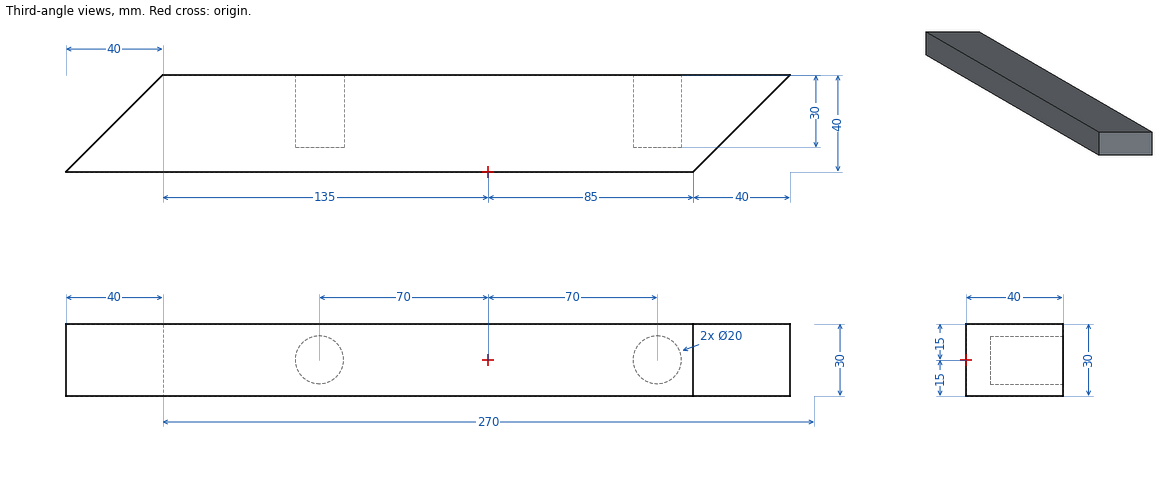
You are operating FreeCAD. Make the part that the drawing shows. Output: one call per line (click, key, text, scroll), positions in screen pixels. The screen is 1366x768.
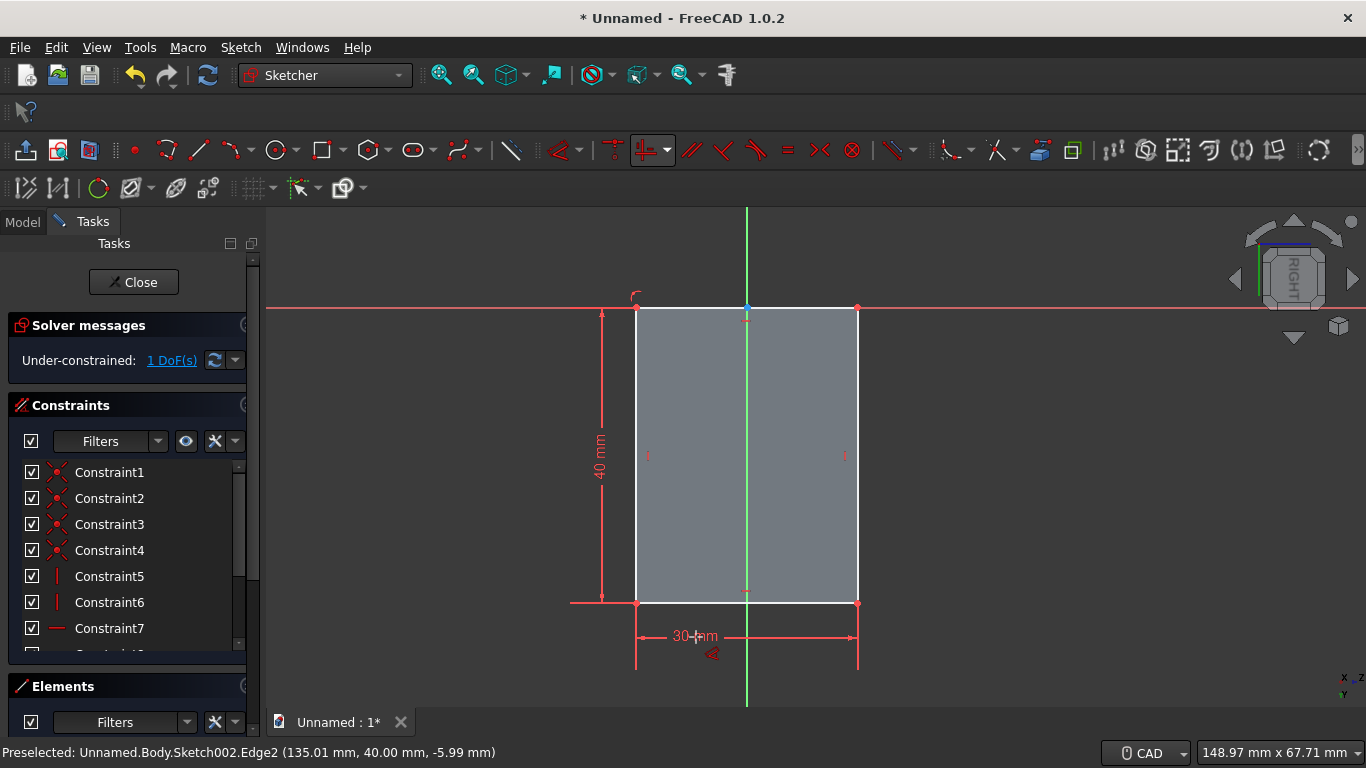
click(636, 308)
click(692, 274)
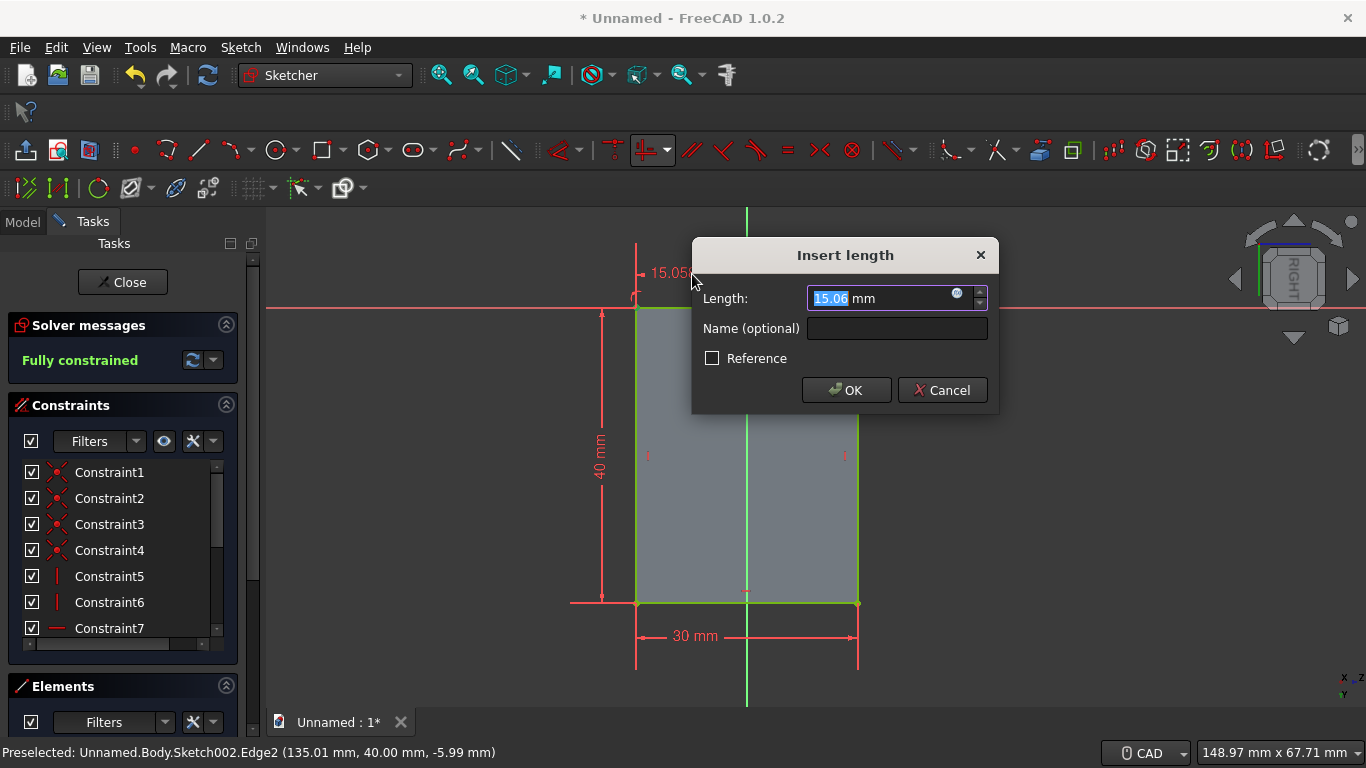
text(15)
key(Return)
key(Escape)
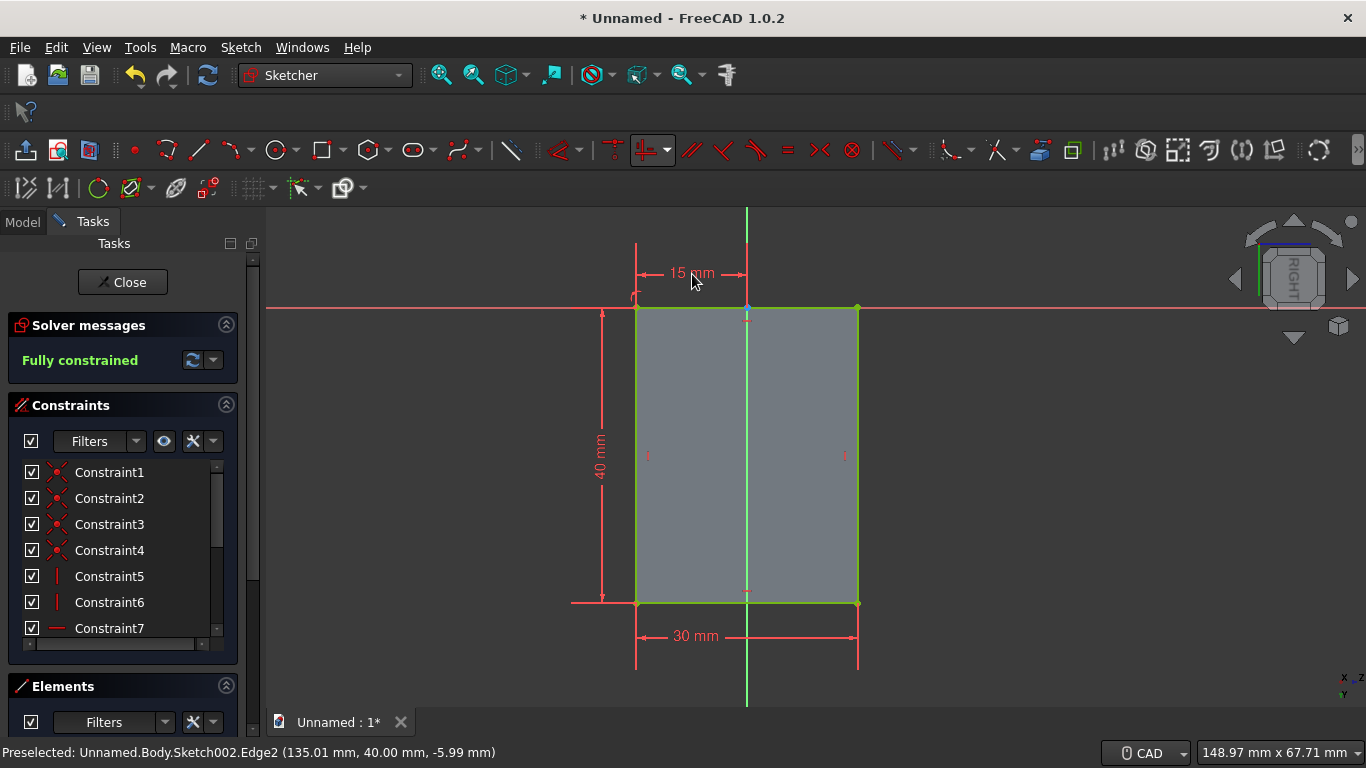
click(123, 282)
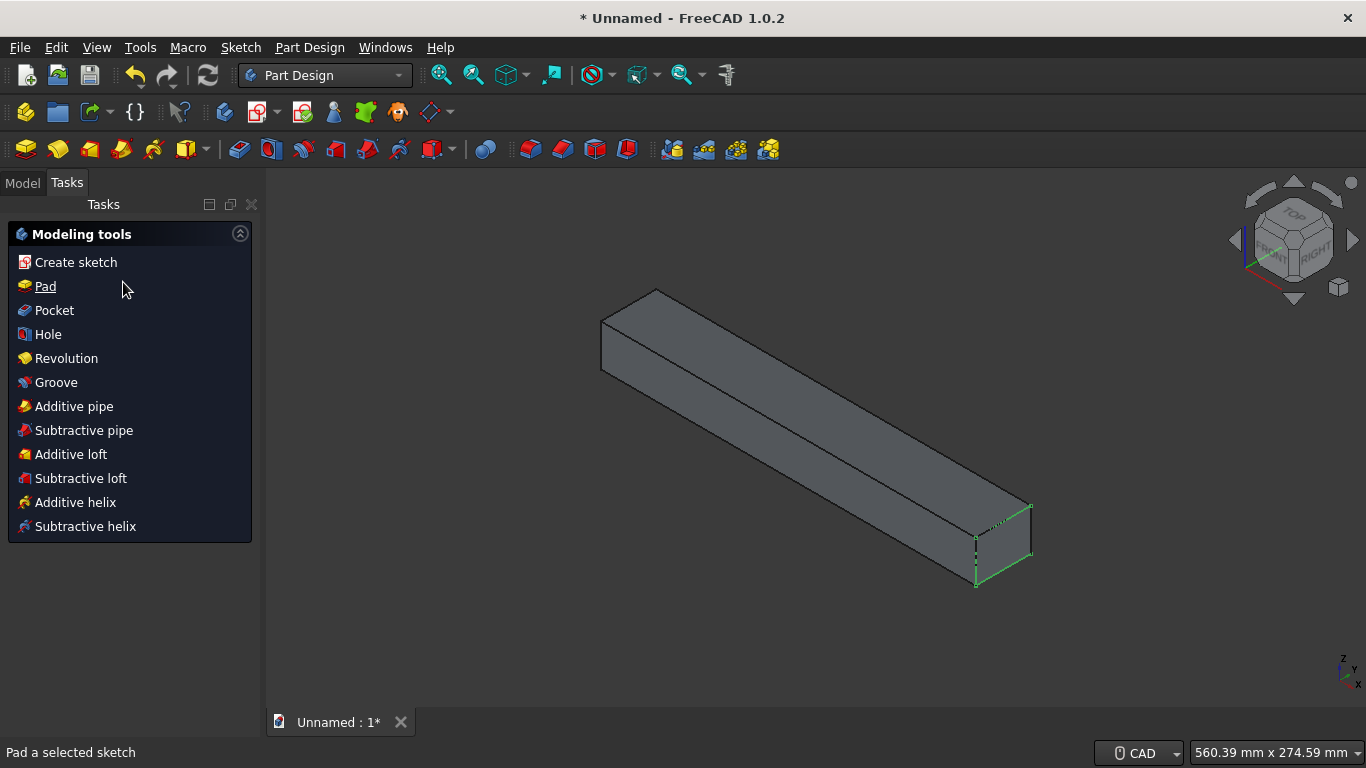
click(240, 150)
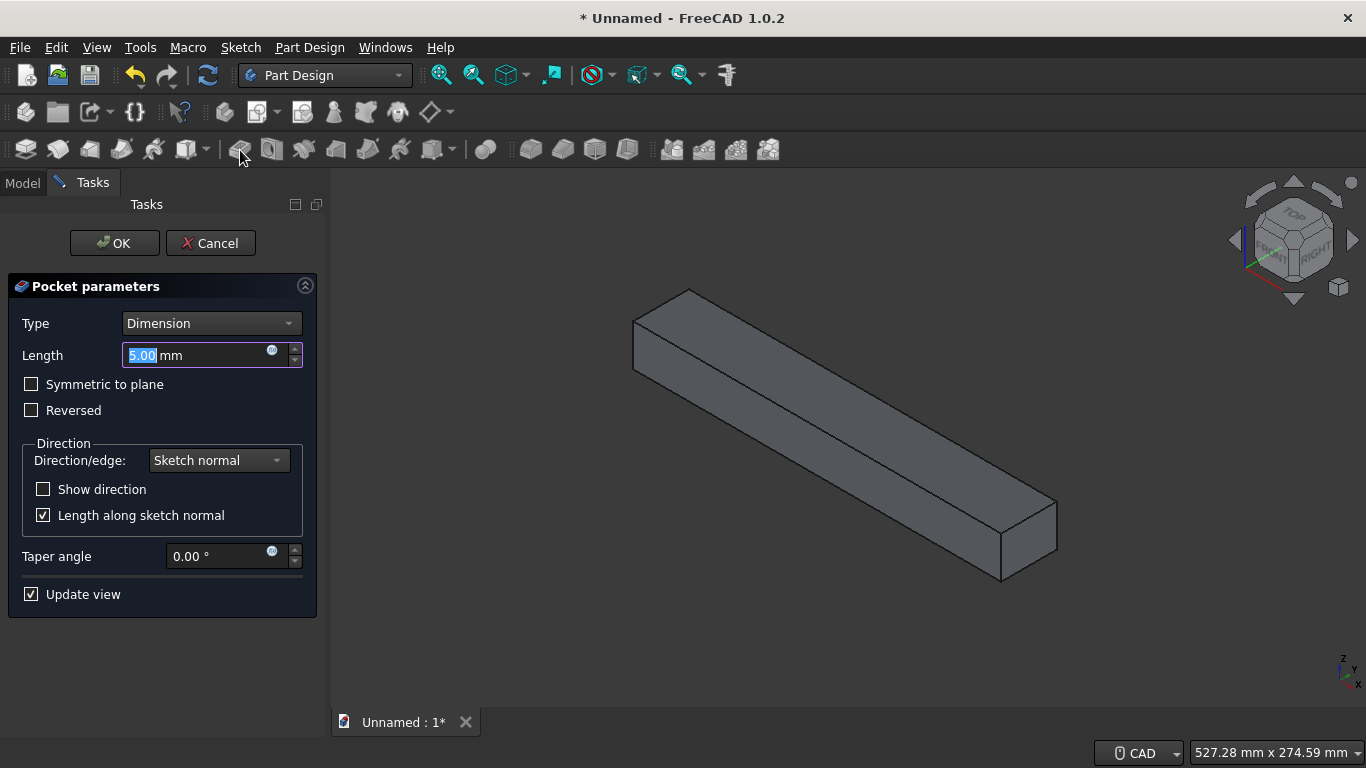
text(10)
key(Tab)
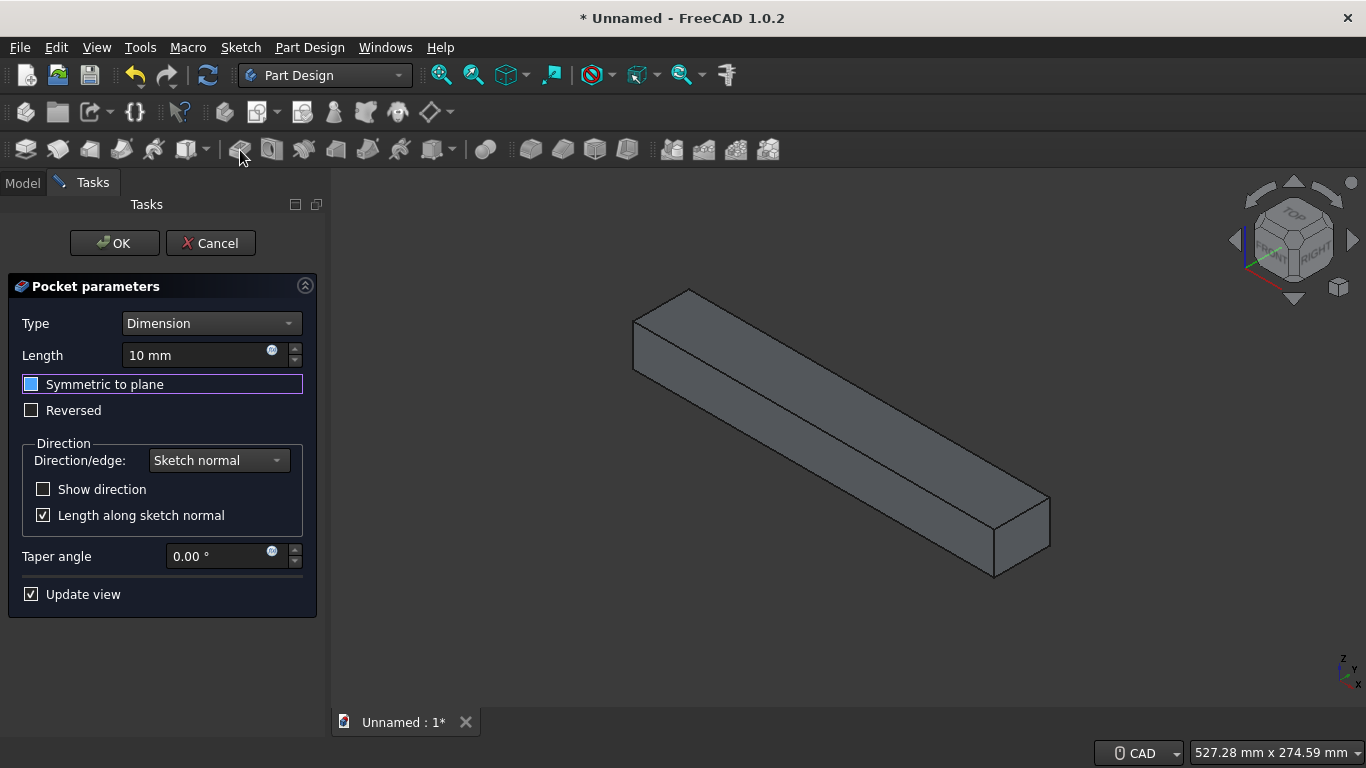
click(115, 243)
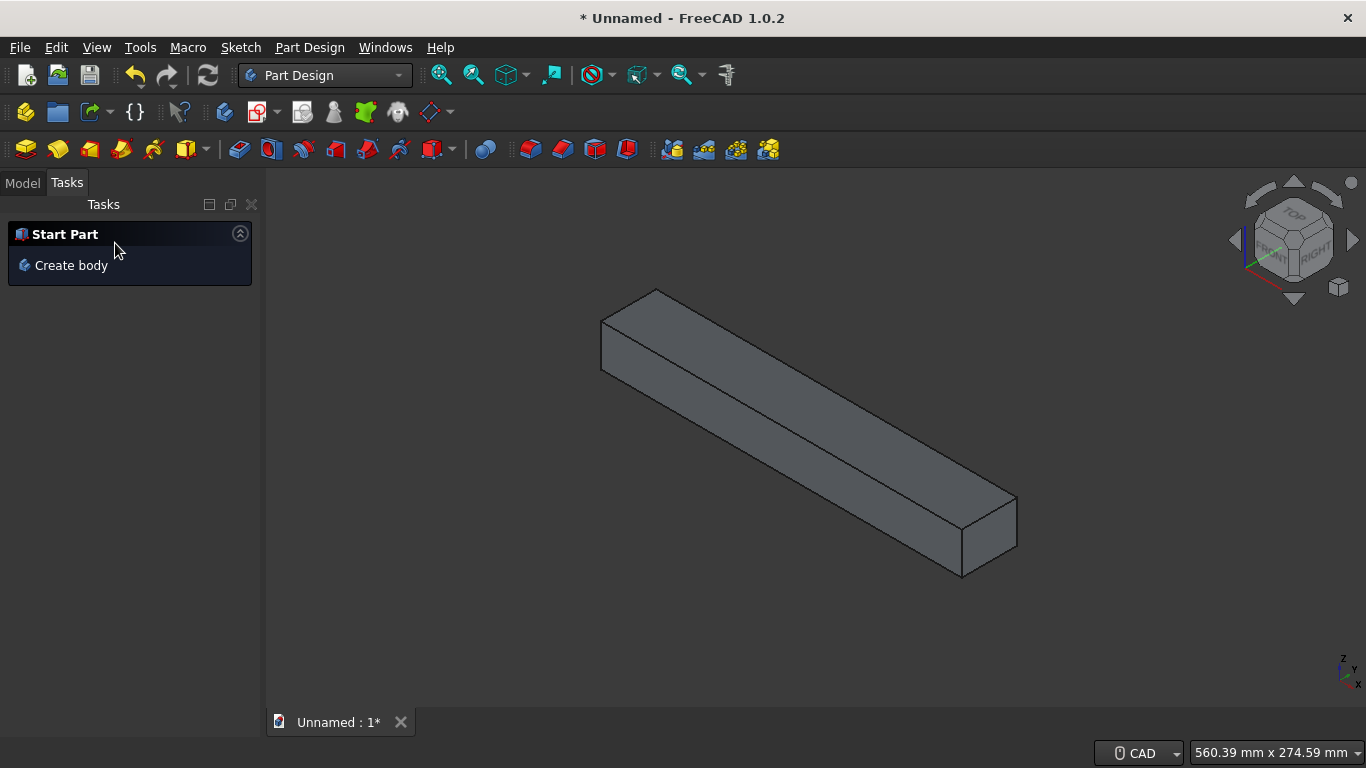
click(912, 468)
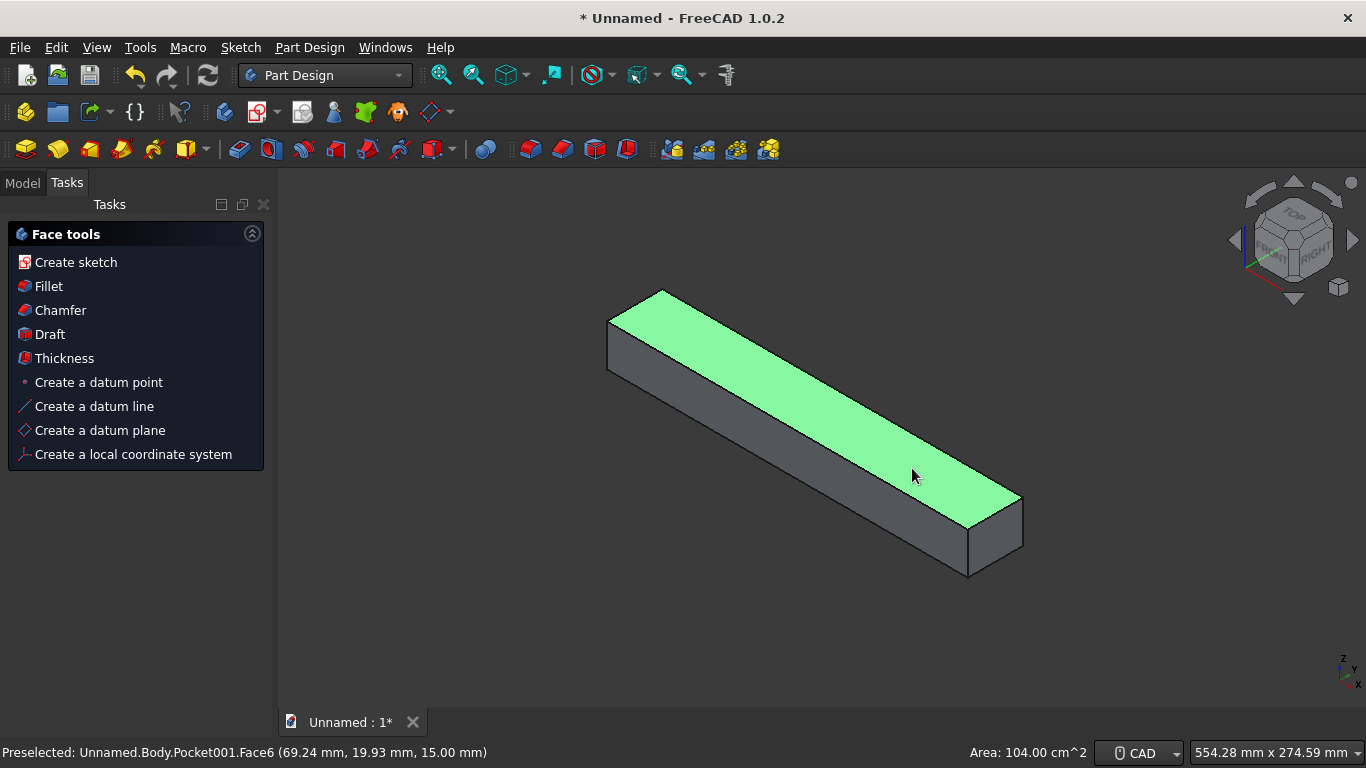
click(258, 112)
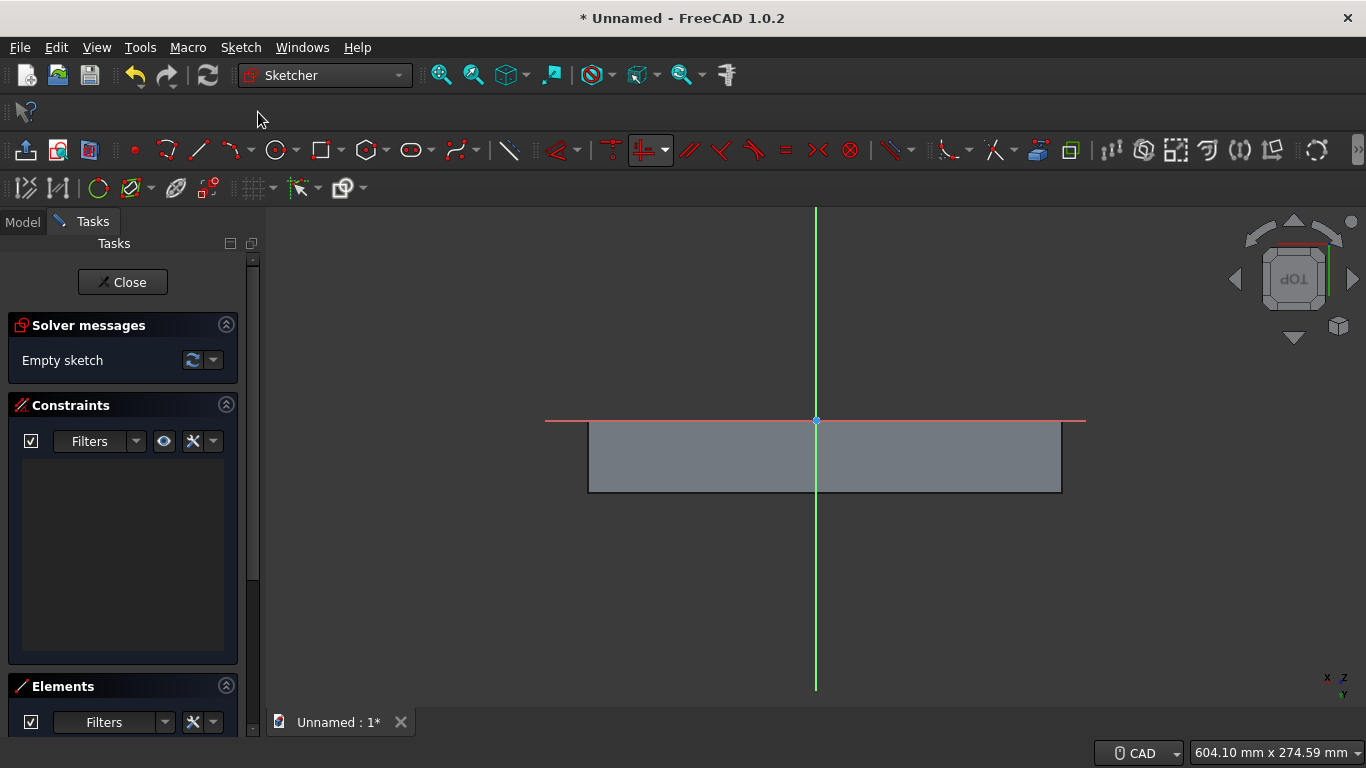
scroll(585, 457, up, 7)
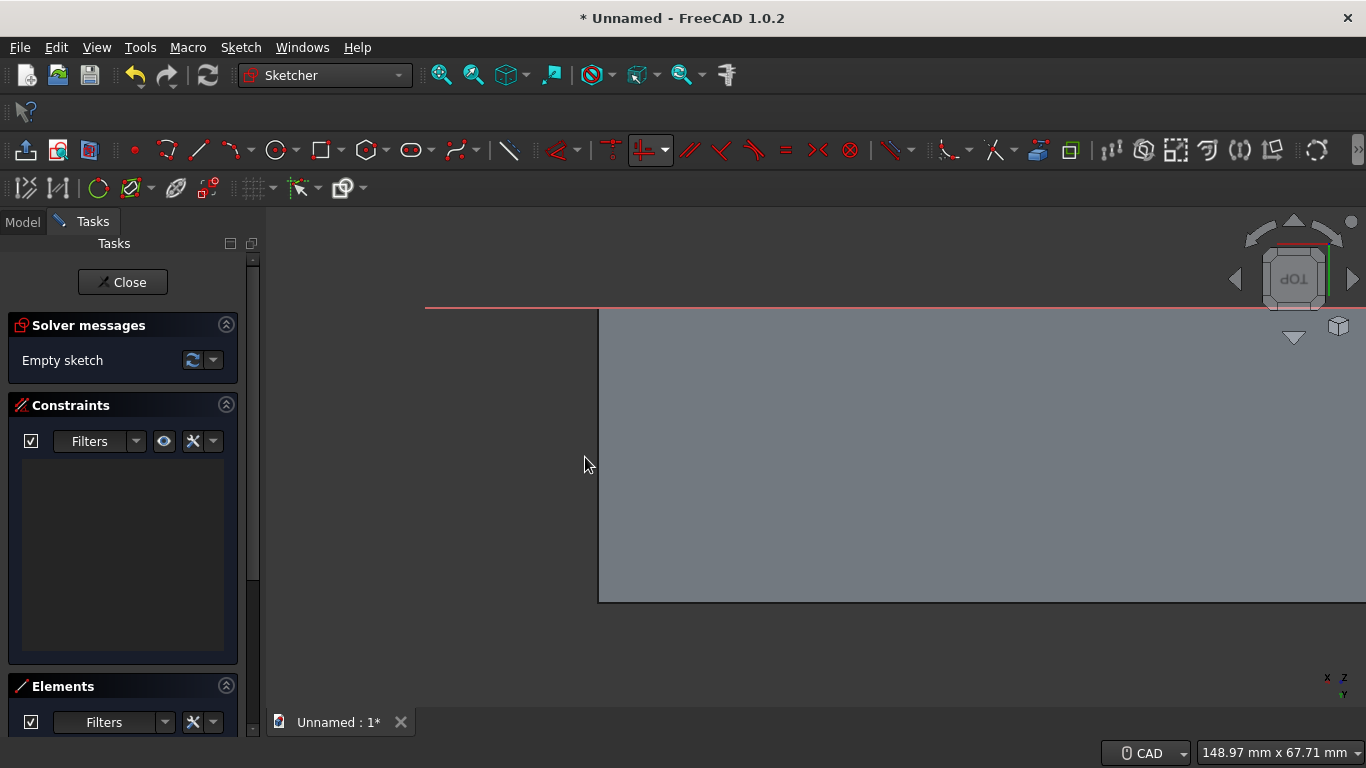
click(168, 150)